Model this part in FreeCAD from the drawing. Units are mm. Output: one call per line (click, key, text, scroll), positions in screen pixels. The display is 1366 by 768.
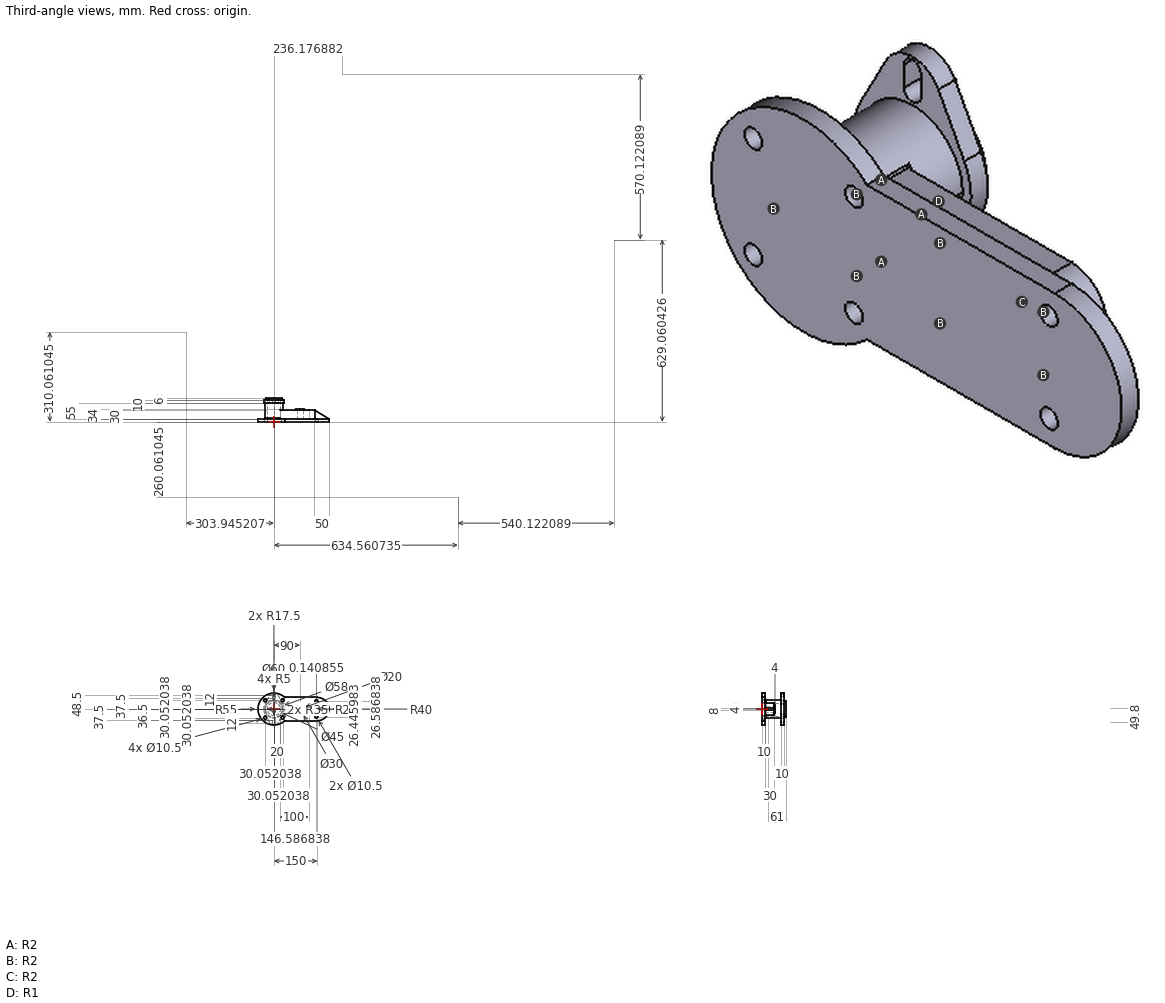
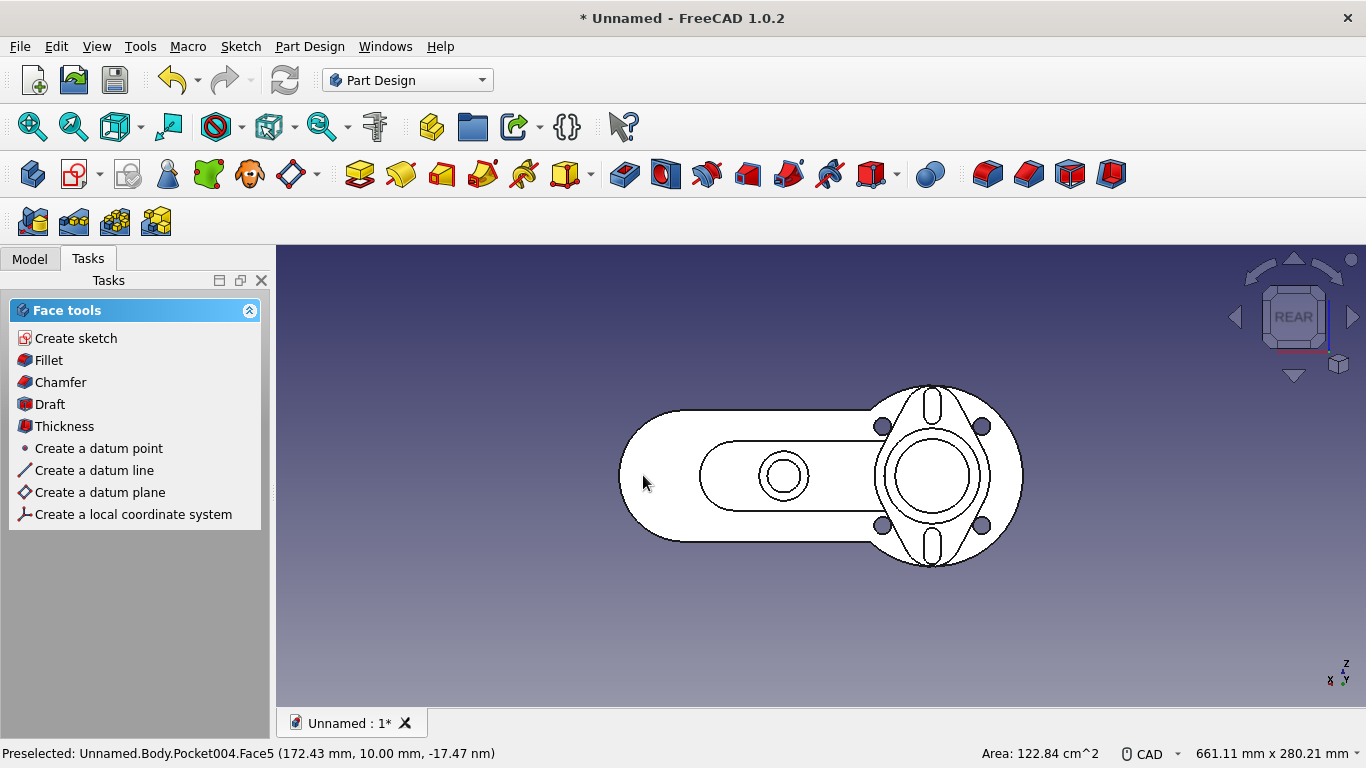
click(74, 174)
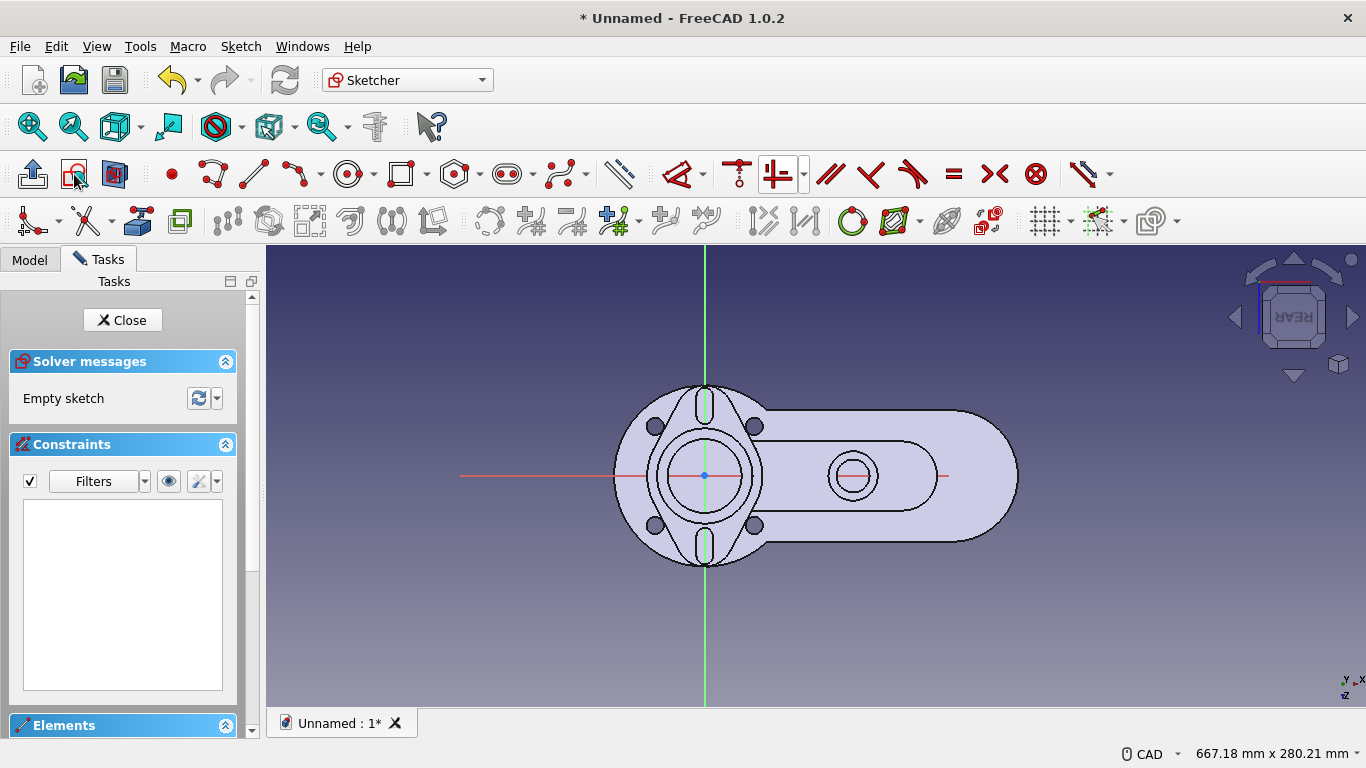
click(115, 174)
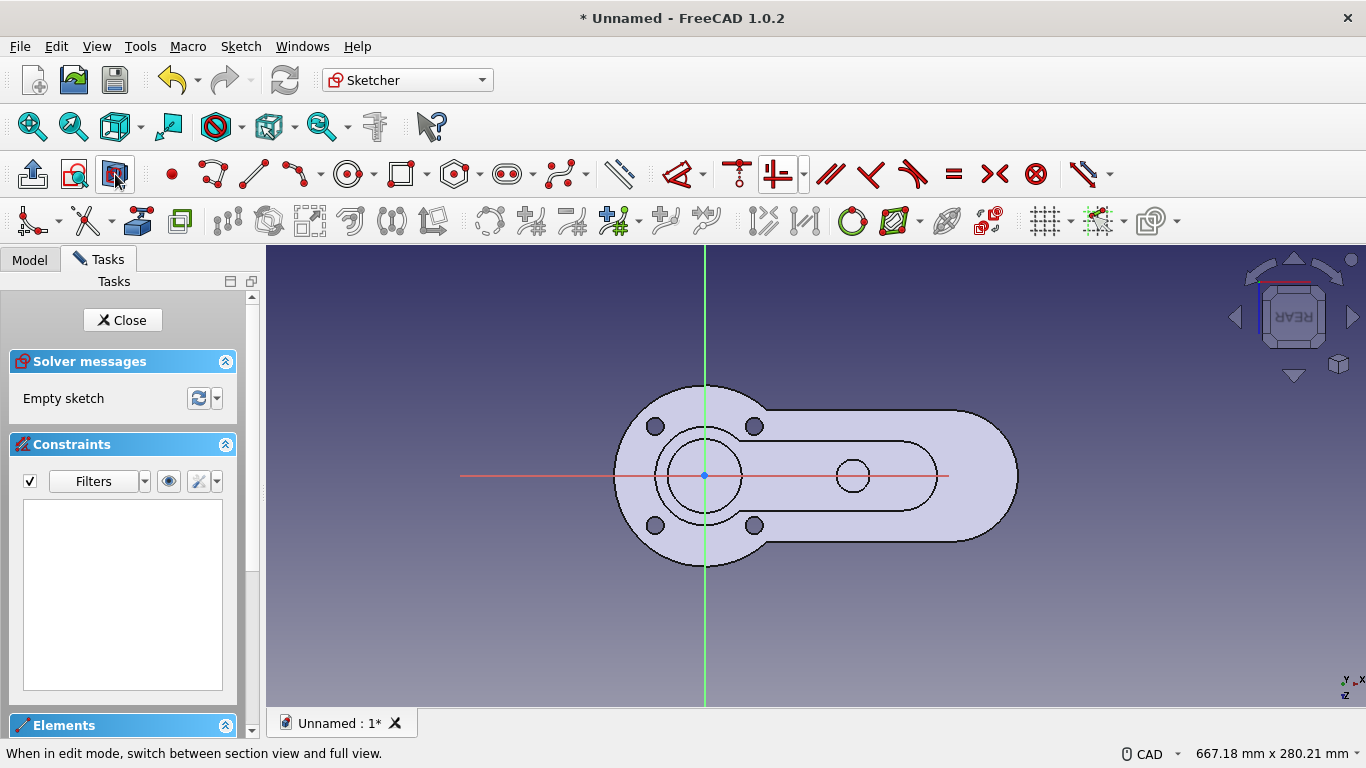
scroll(878, 476, up, 5)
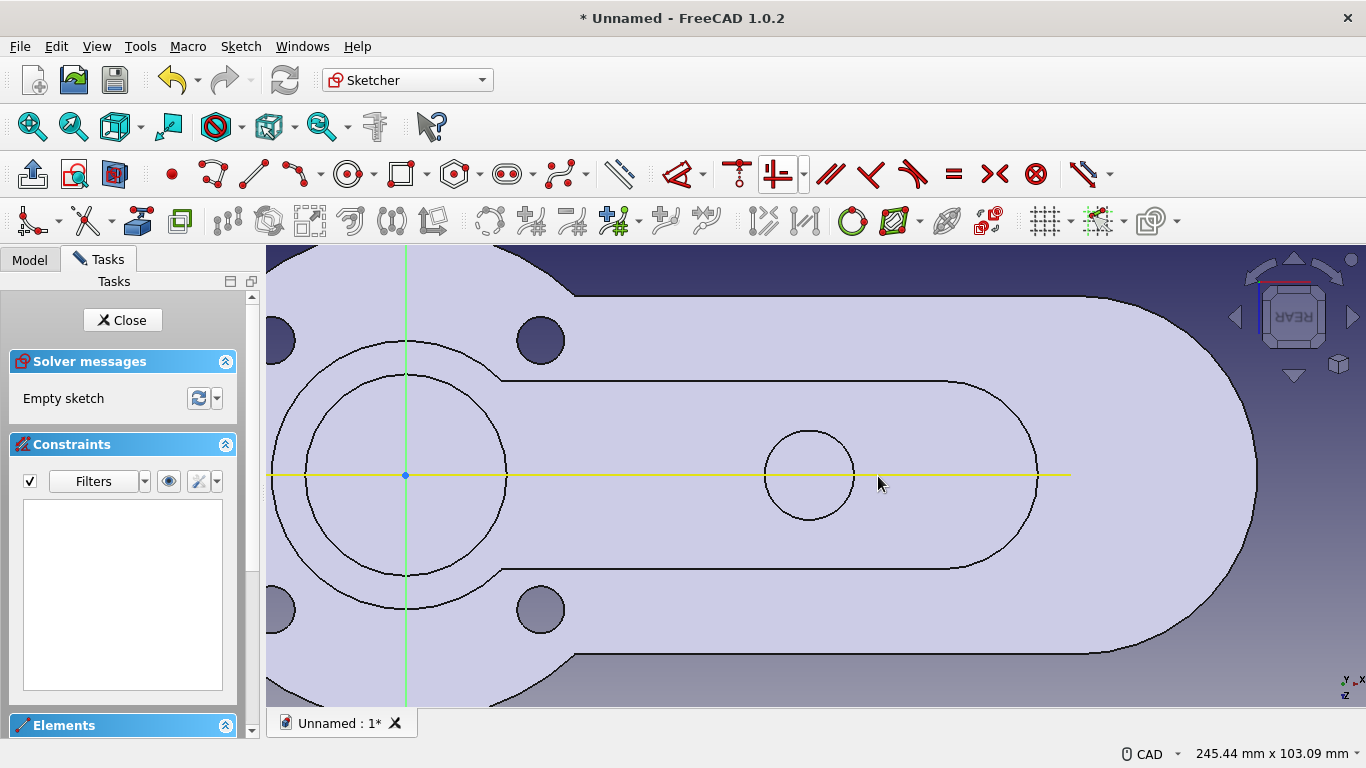
click(348, 174)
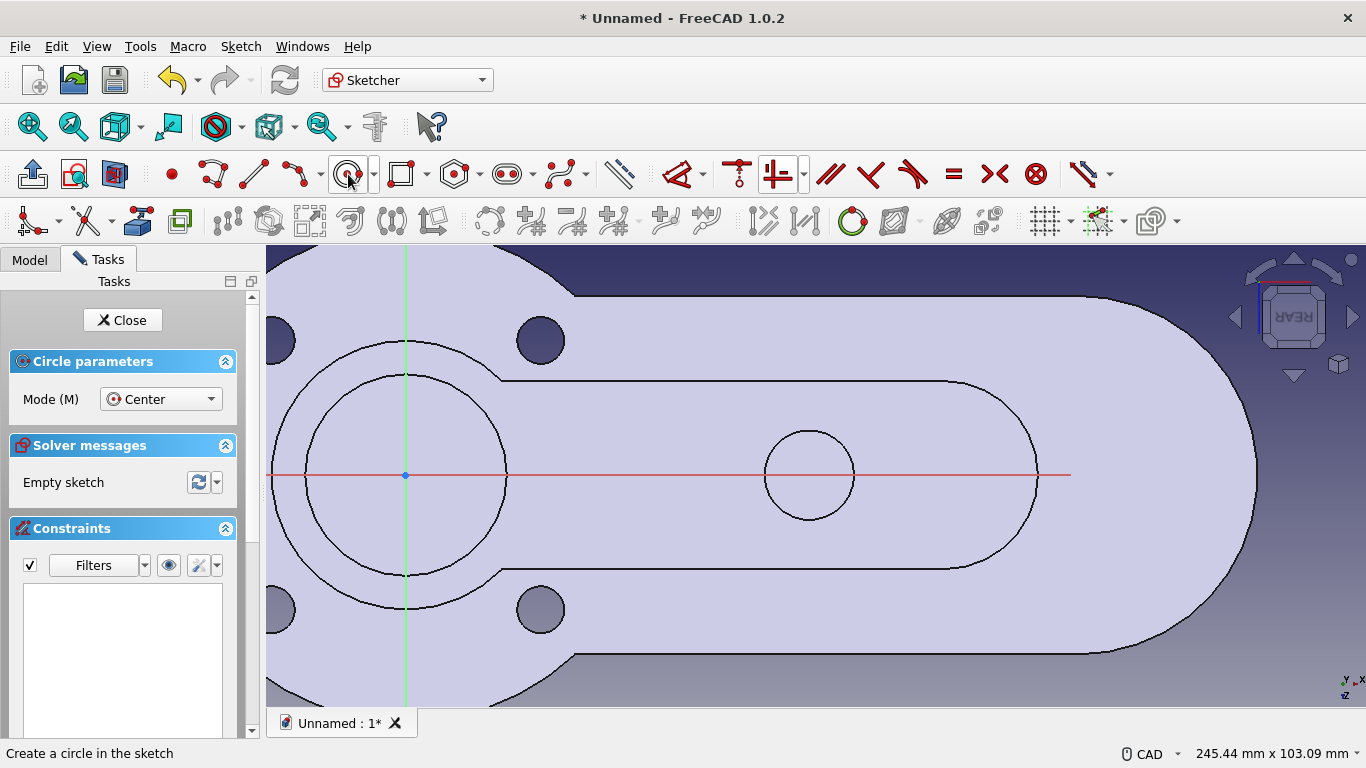
click(1063, 357)
click(1080, 340)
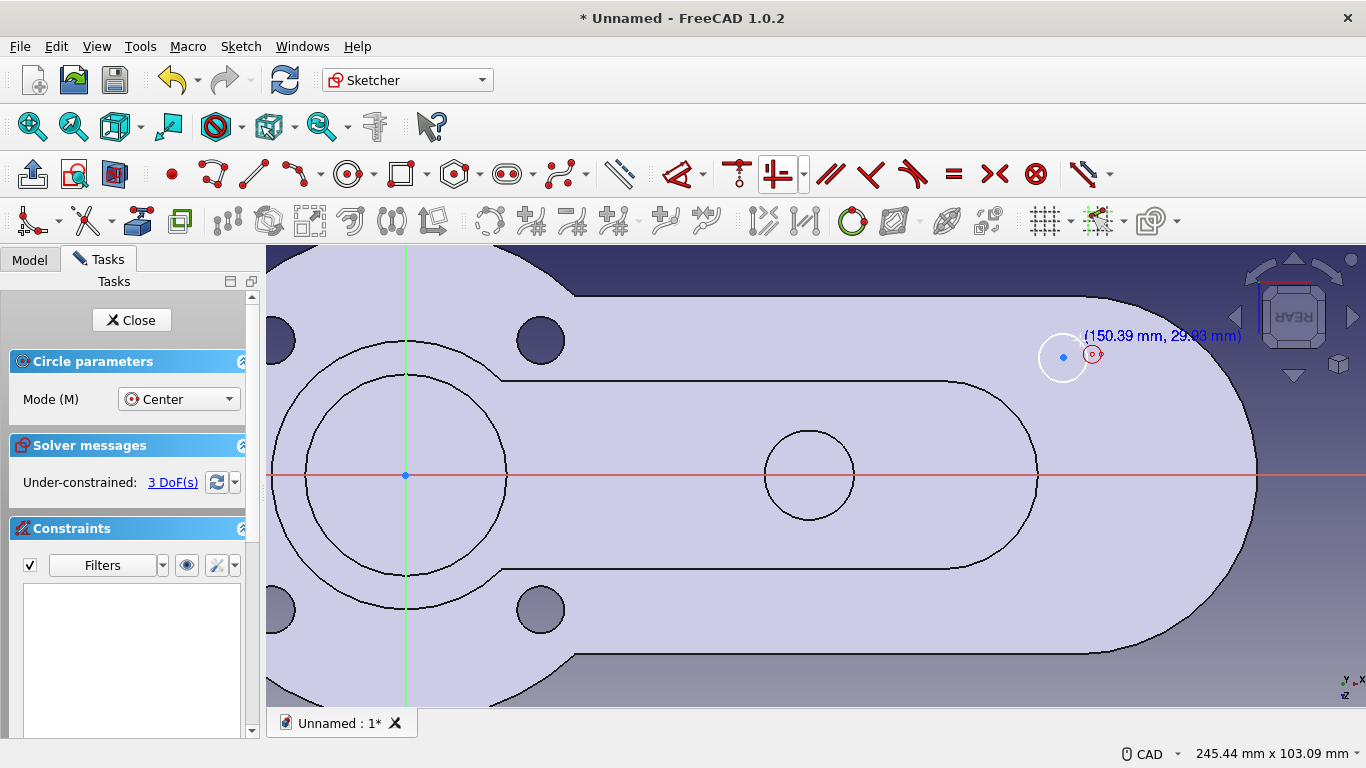
click(1062, 594)
click(1079, 578)
key(Escape)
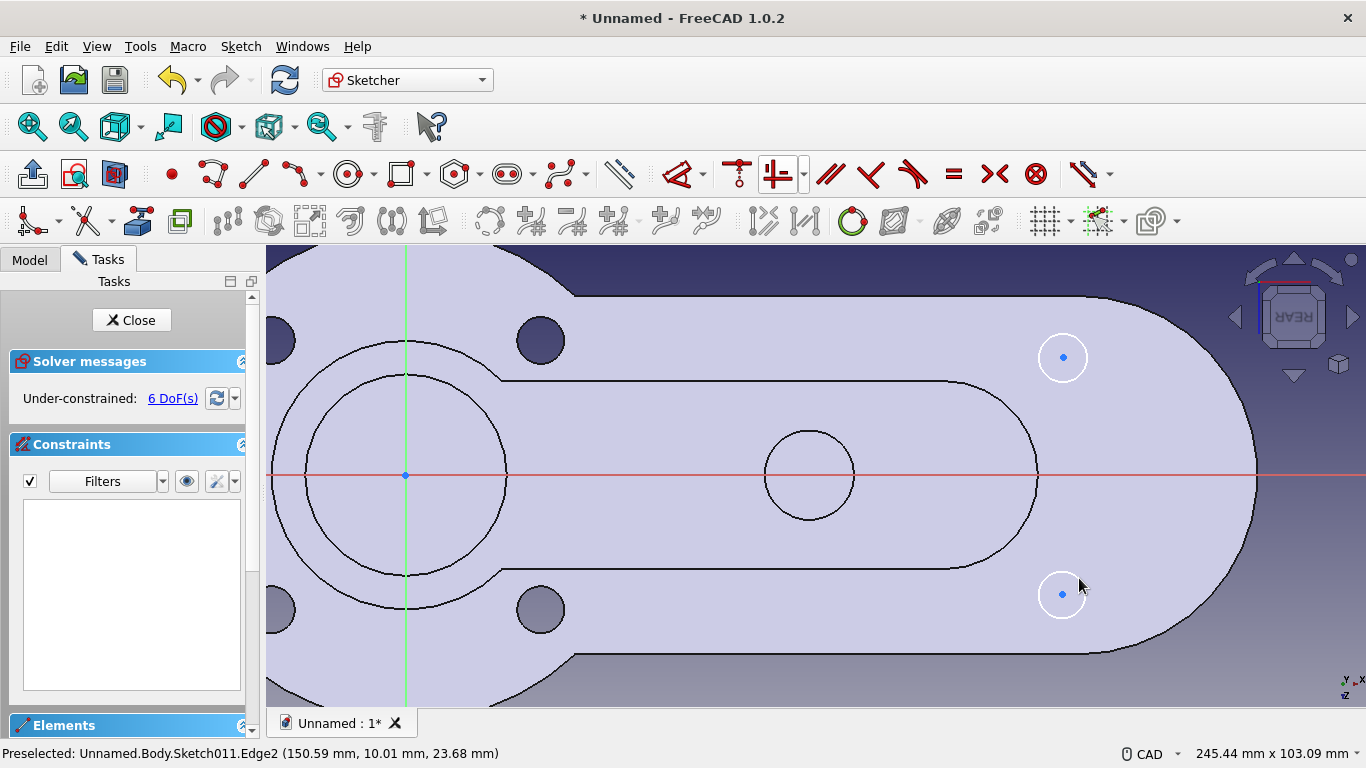
click(1080, 341)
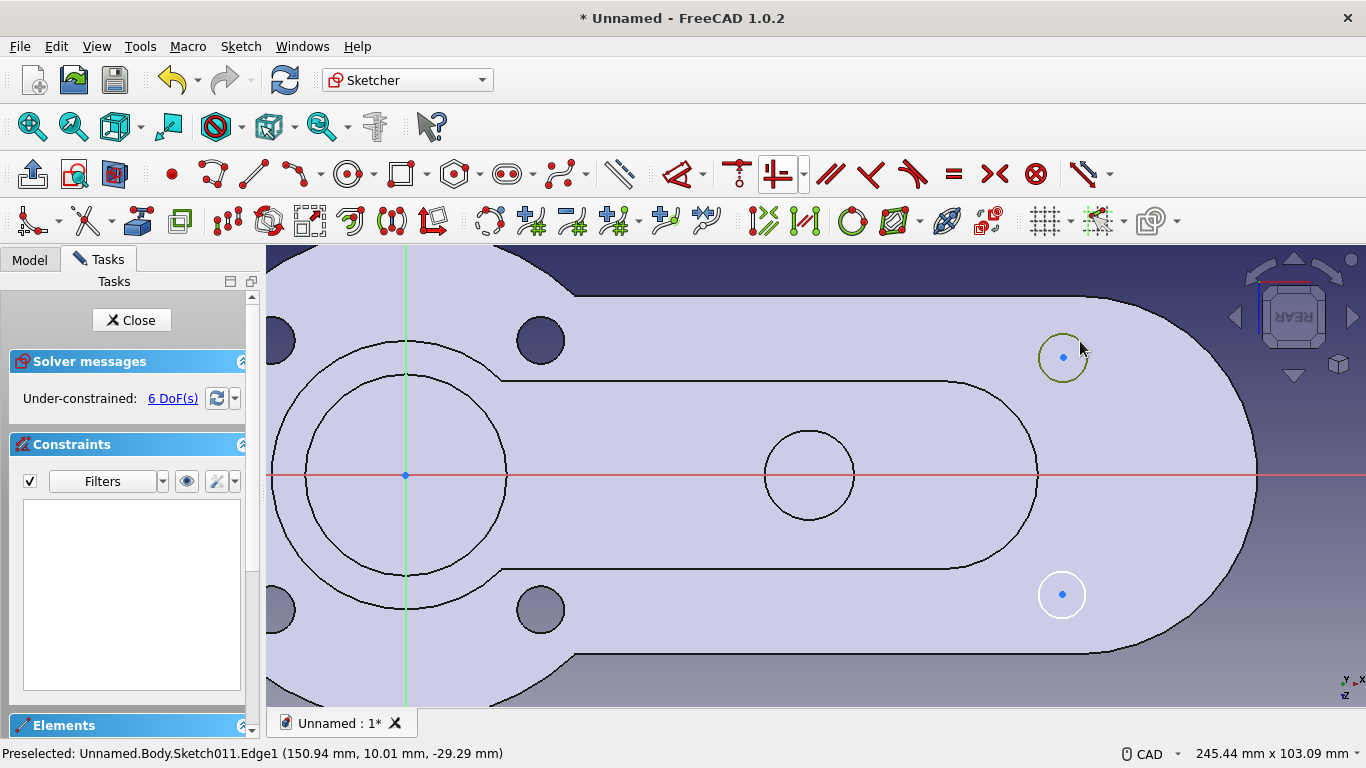
click(1078, 578)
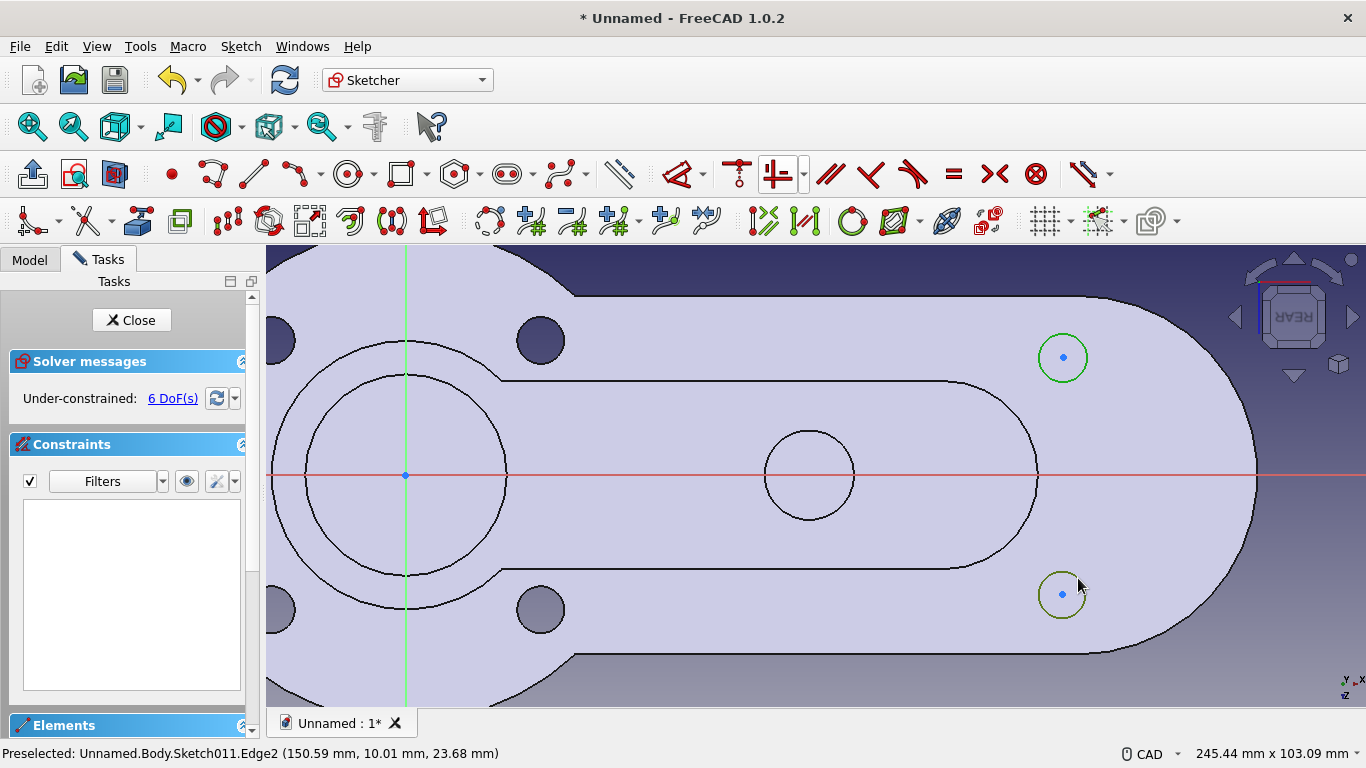
key(e)